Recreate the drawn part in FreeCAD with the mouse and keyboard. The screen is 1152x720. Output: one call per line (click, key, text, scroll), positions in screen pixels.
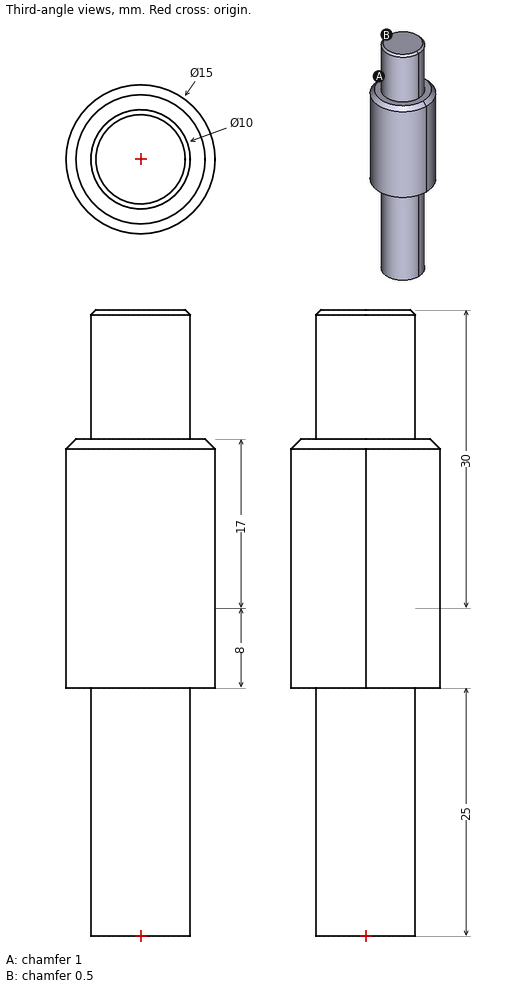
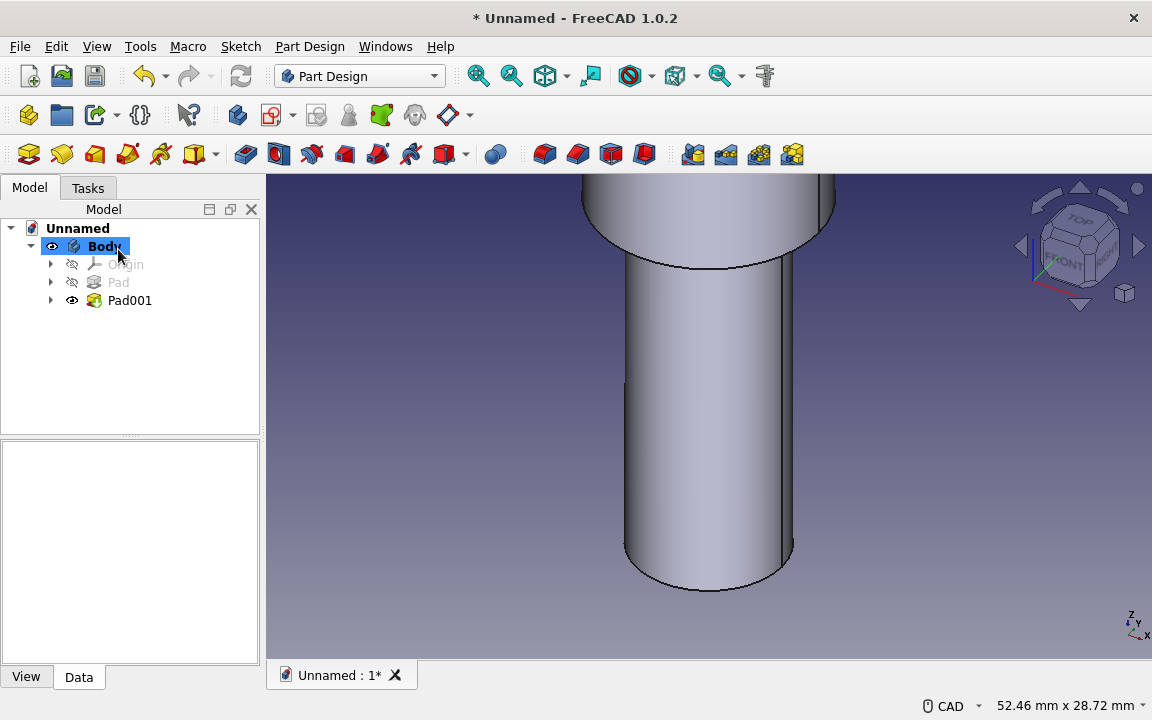
click(479, 76)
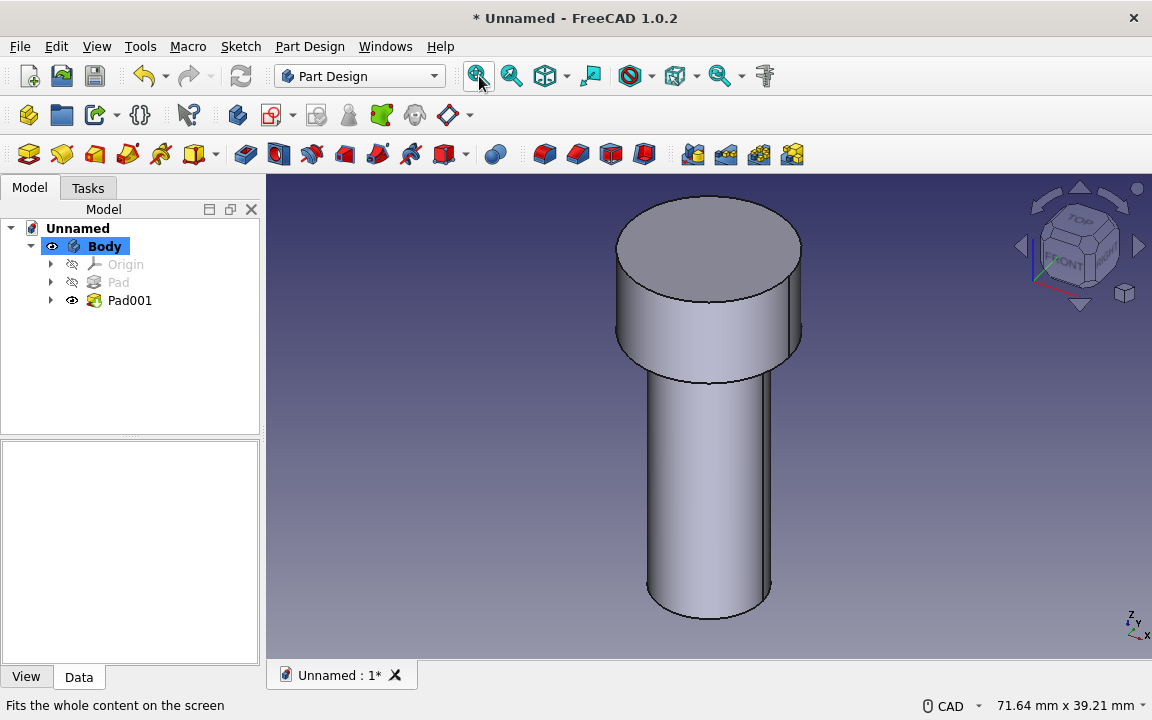
click(709, 248)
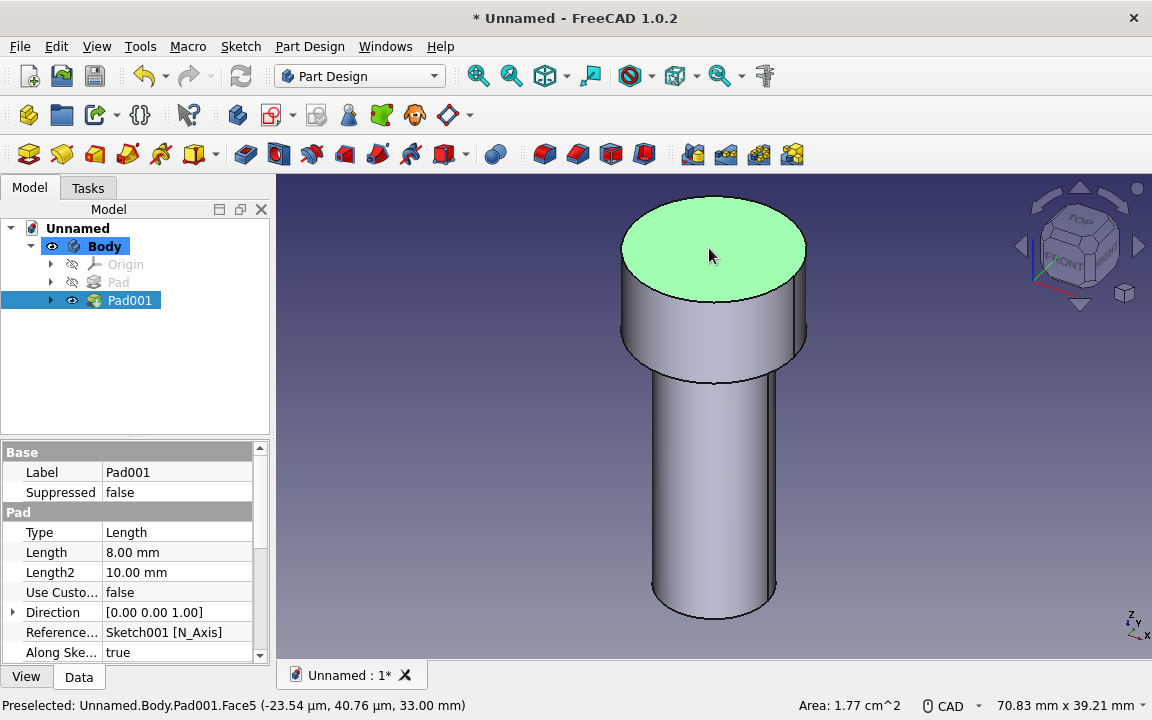
click(270, 116)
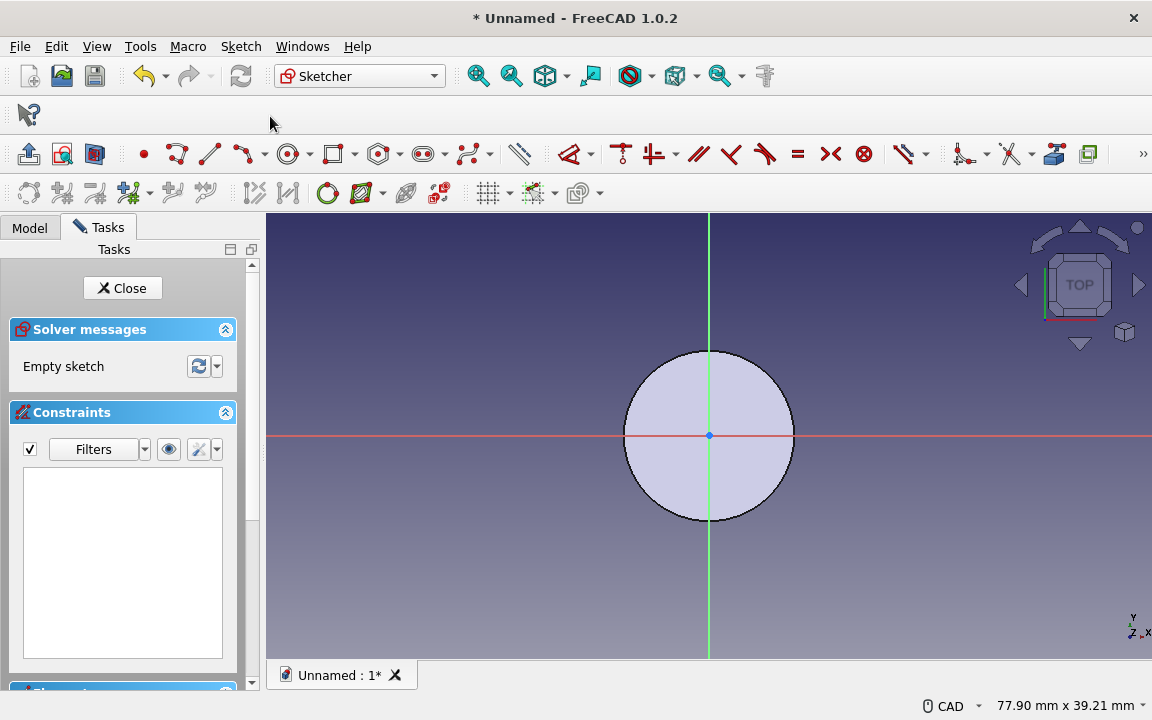
scroll(765, 436, up, 4)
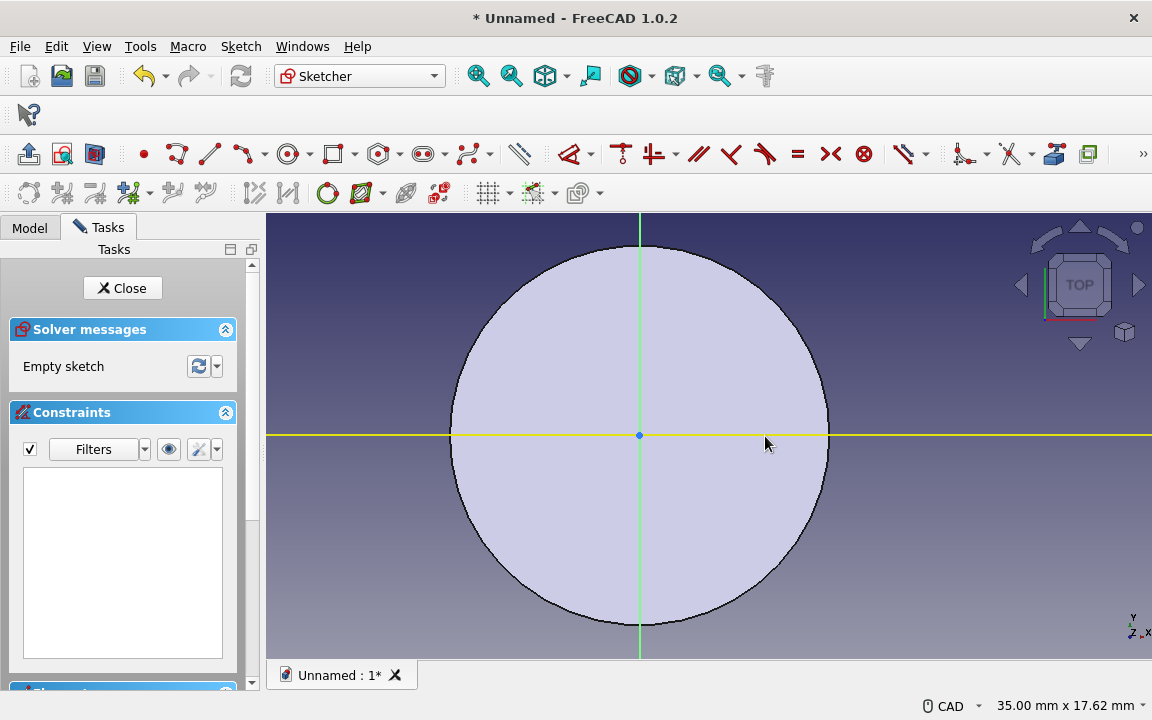
key(g)
key(c)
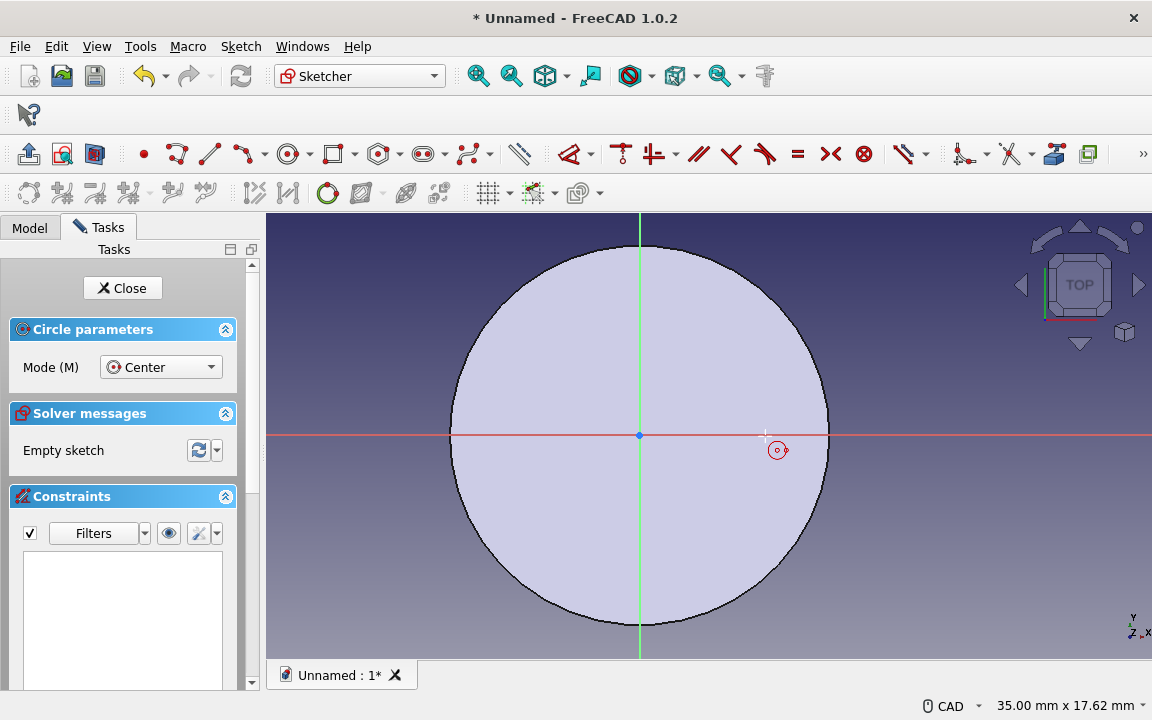
click(640, 435)
click(729, 346)
key(Escape)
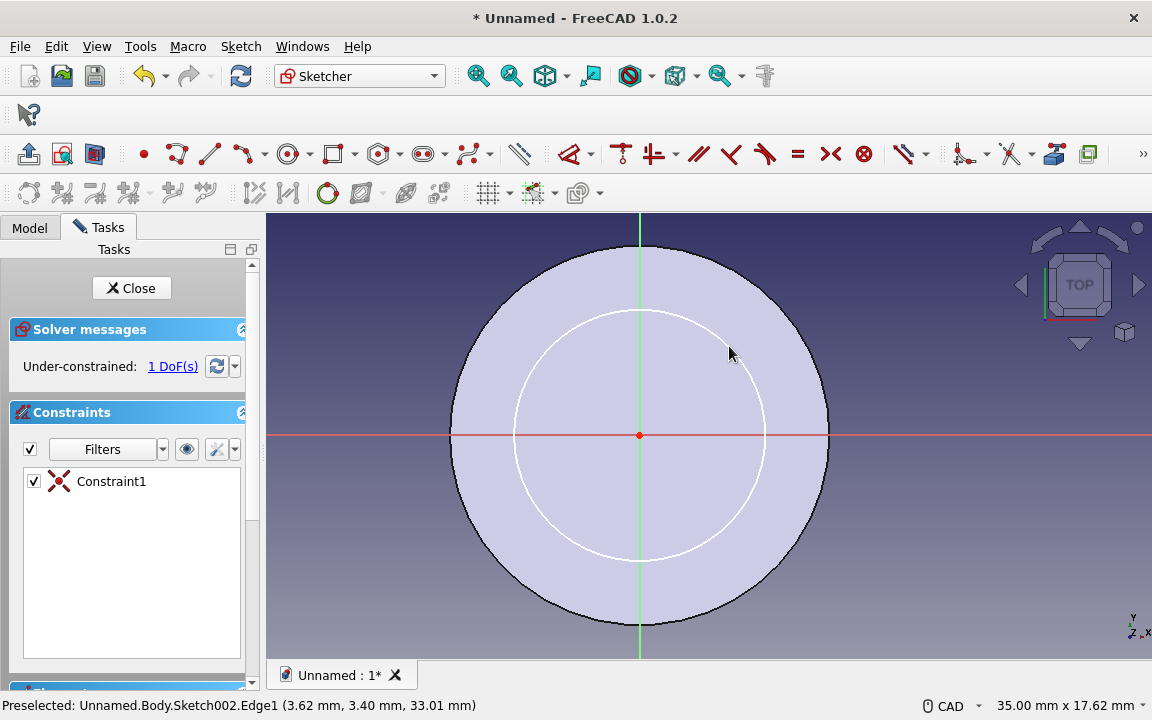
key(d)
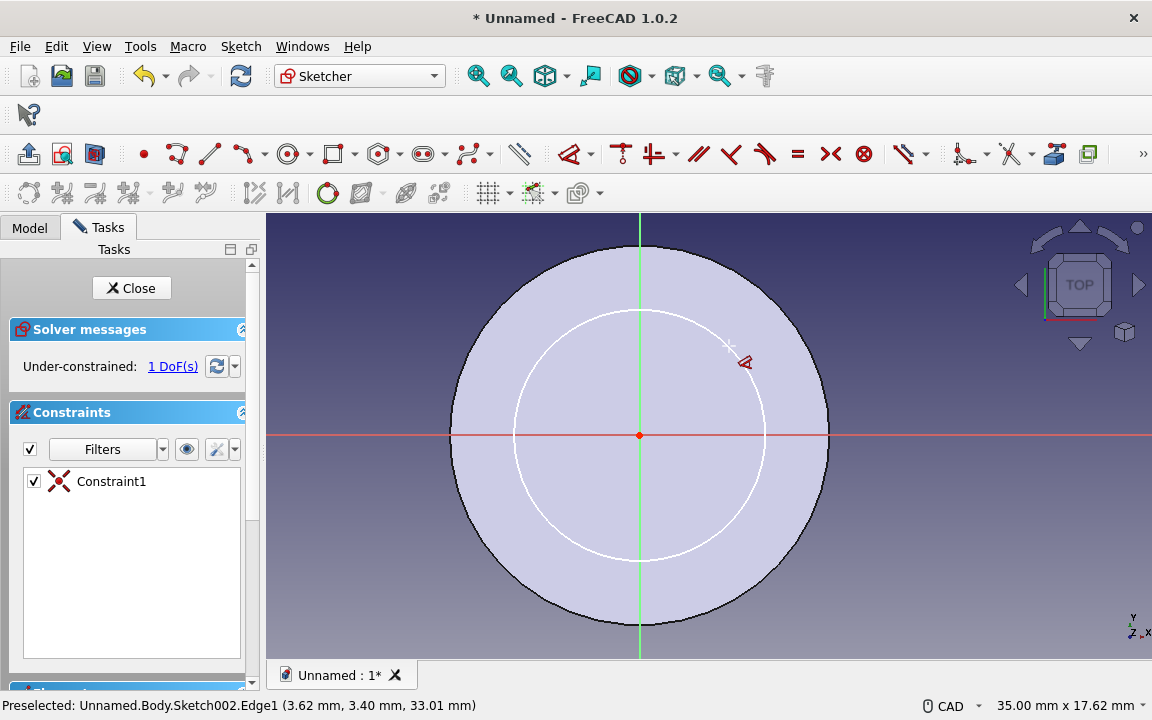
click(728, 346)
click(750, 323)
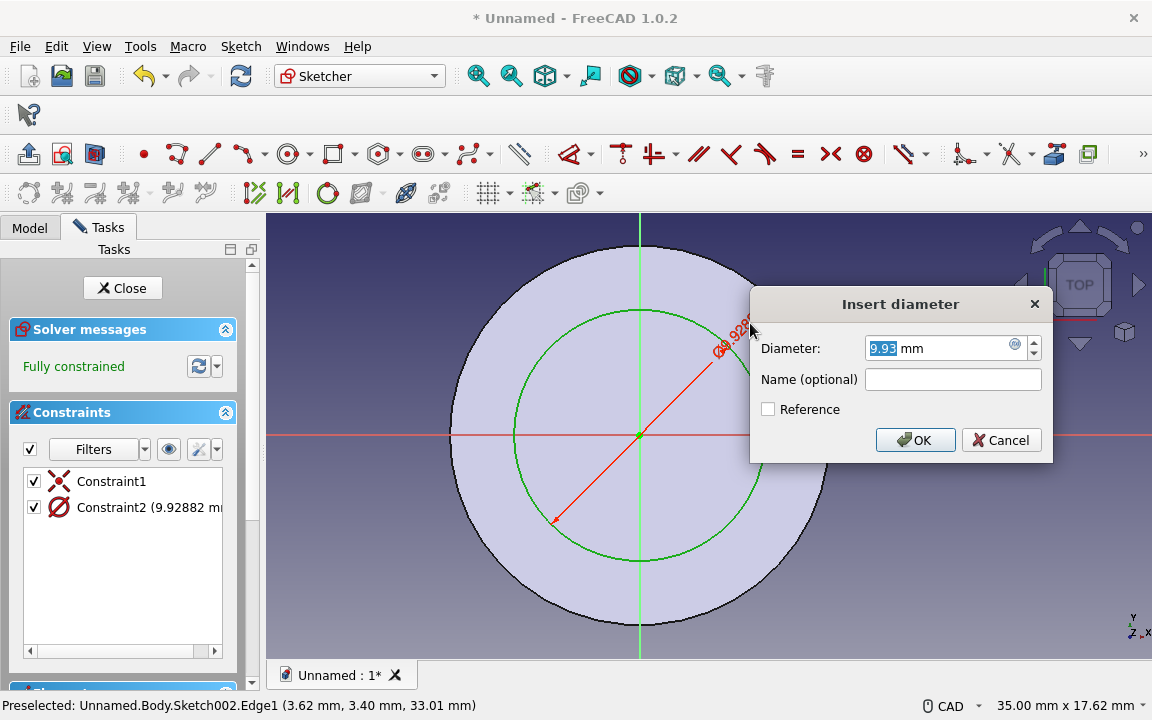
text(10)
key(Return)
key(Escape)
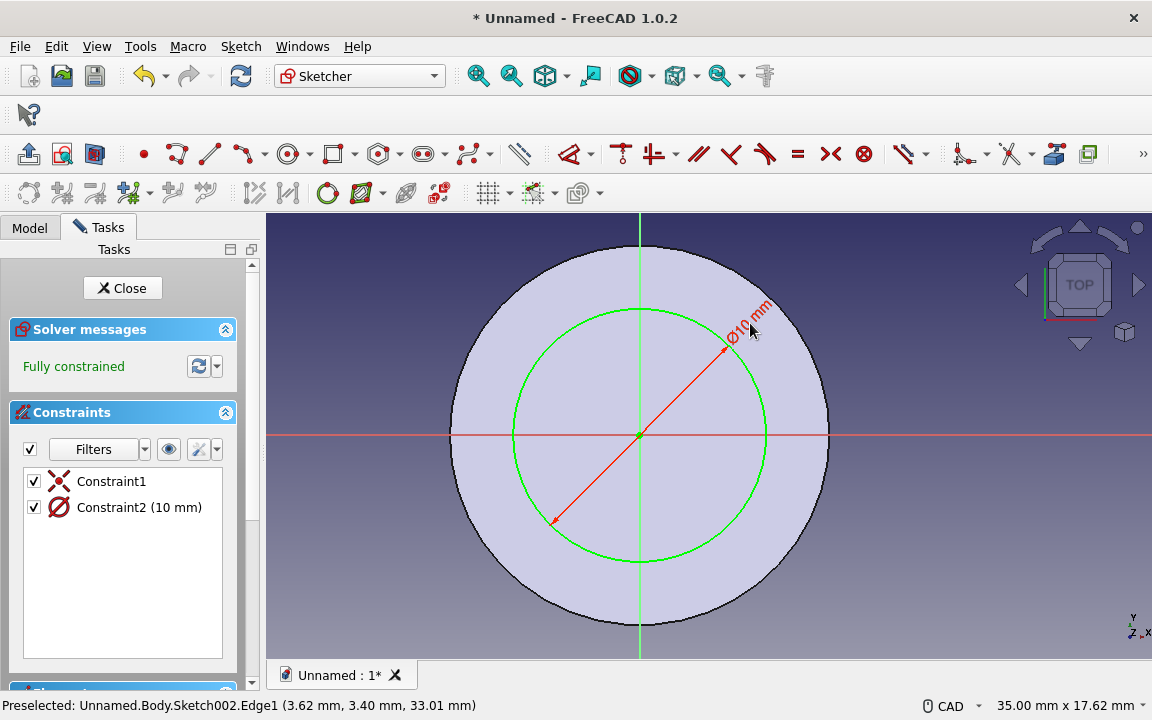
click(123, 288)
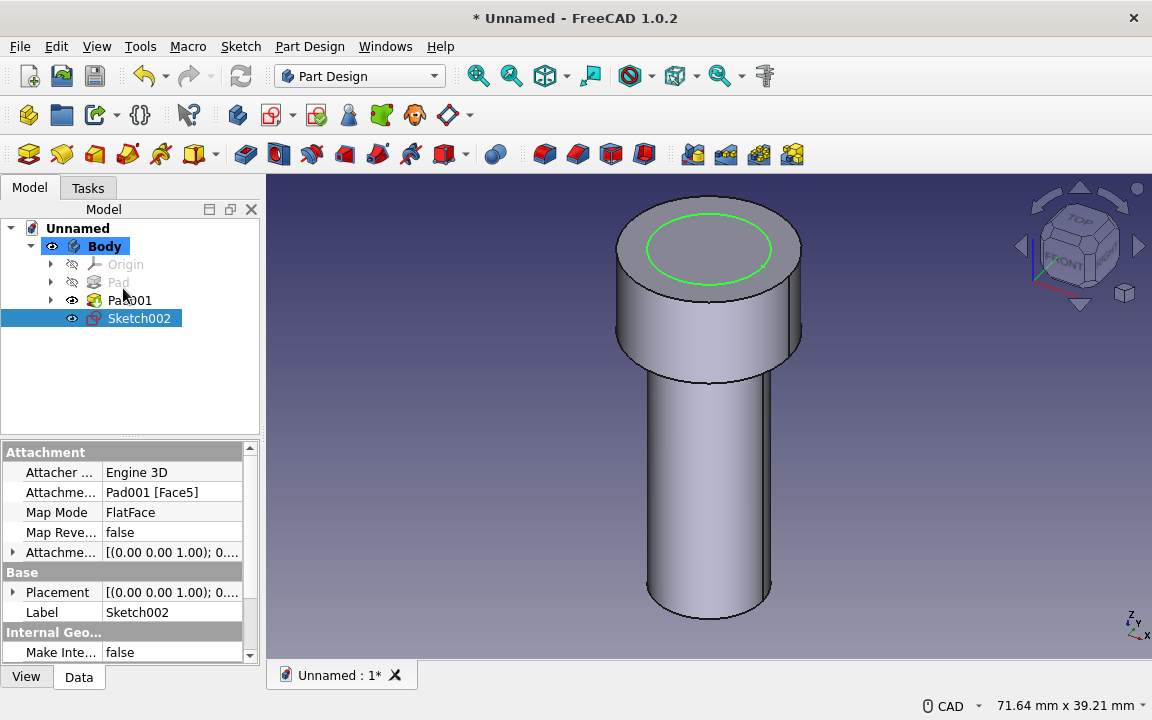
click(29, 154)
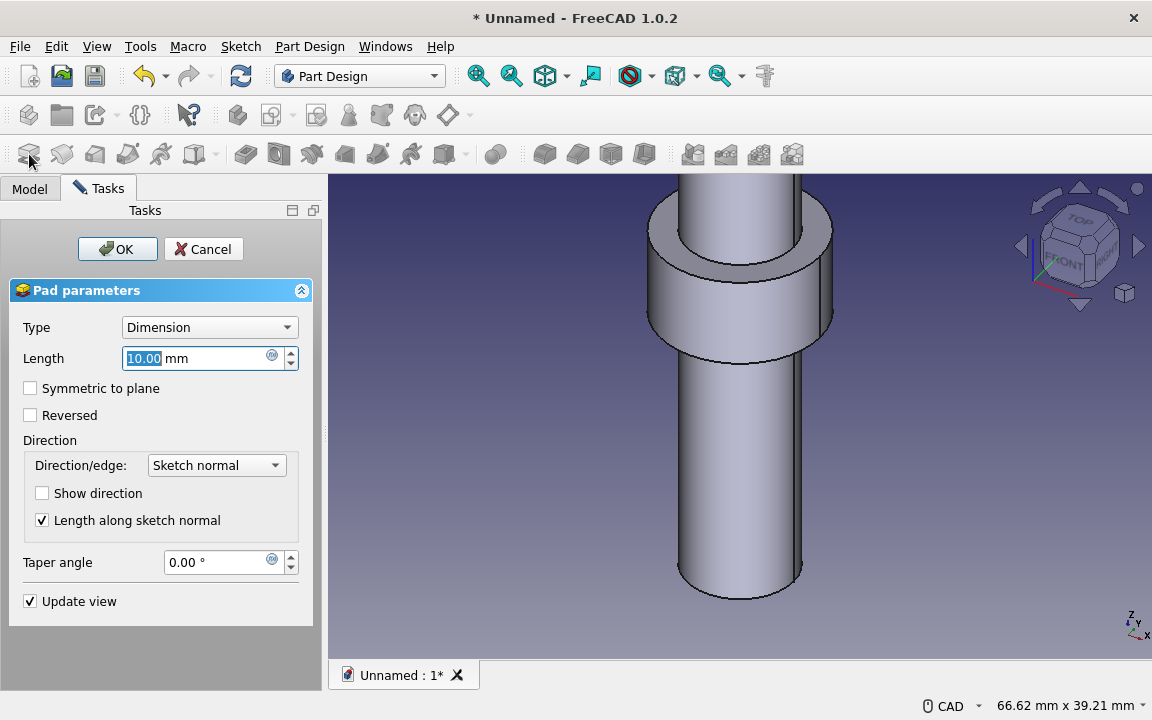
text(30)
key(Tab)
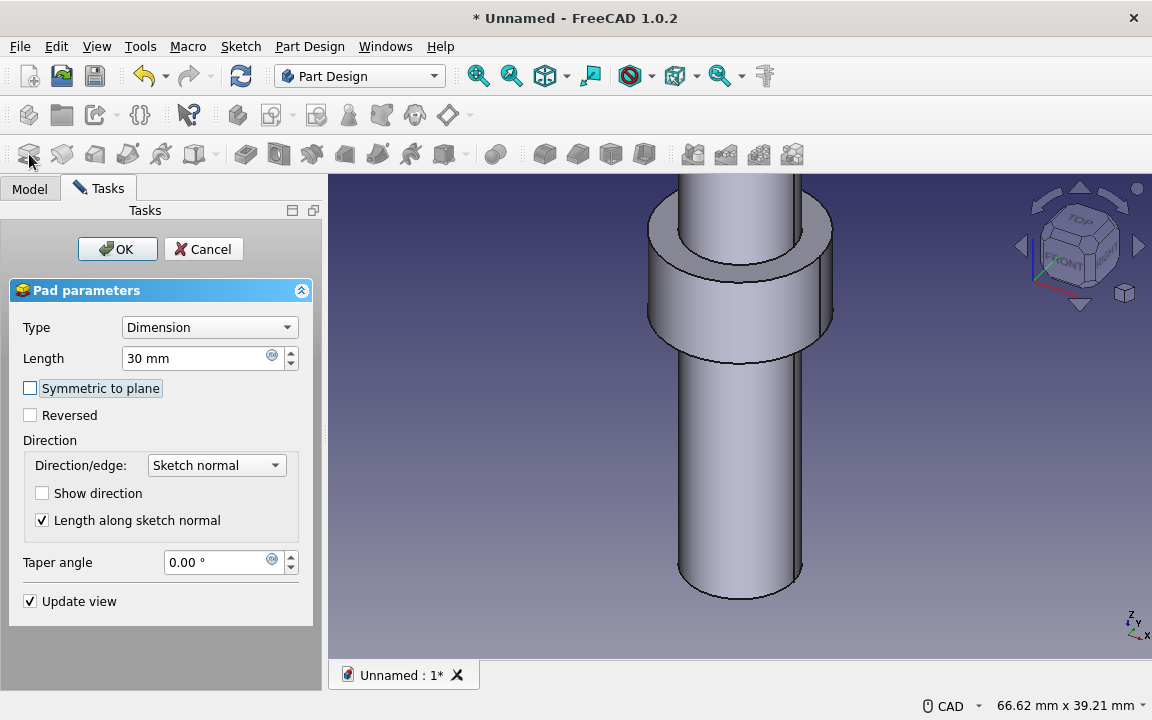
click(118, 249)